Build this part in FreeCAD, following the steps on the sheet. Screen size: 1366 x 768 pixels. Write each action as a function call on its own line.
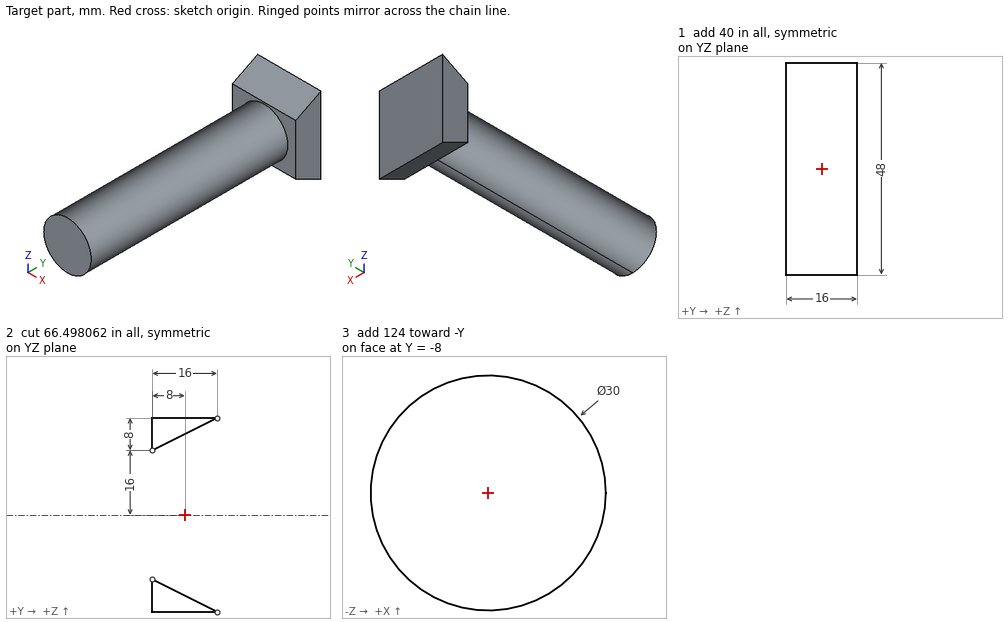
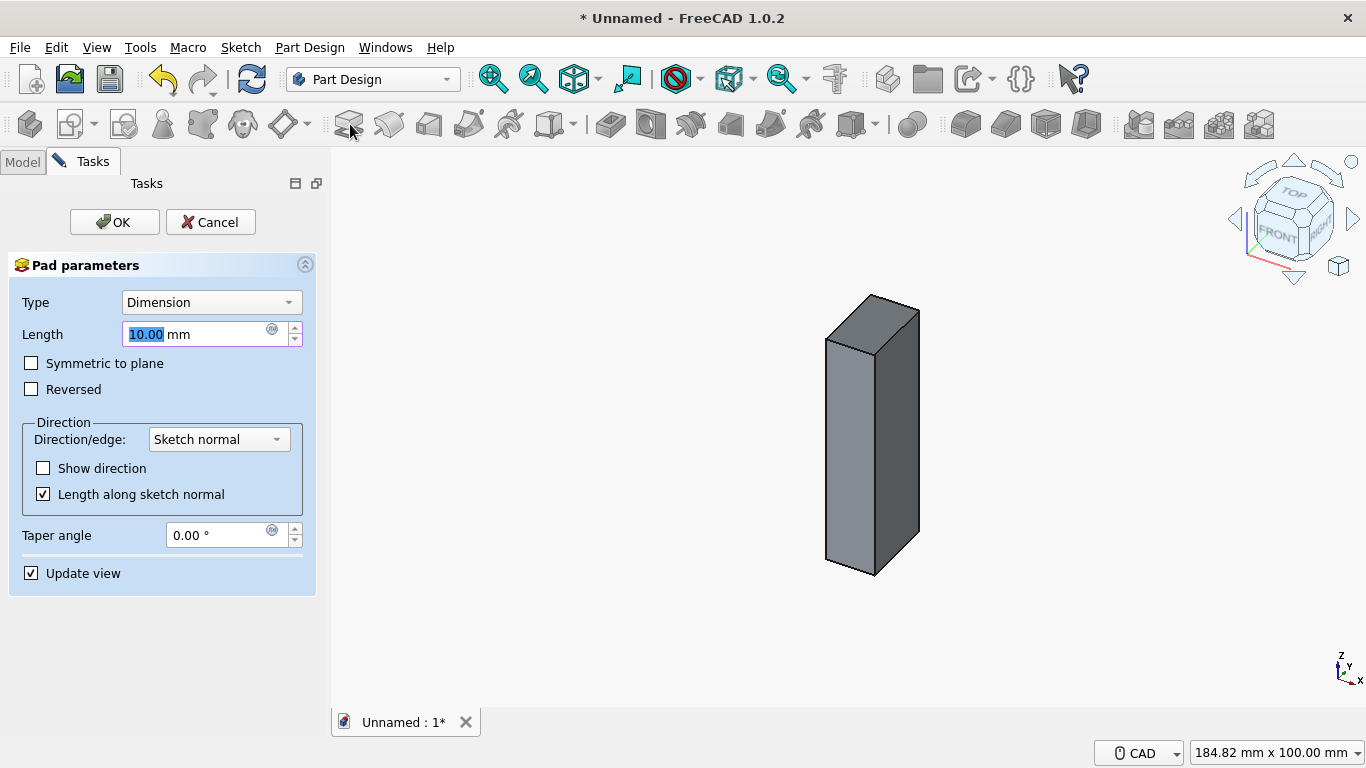
text(40)
key(Tab)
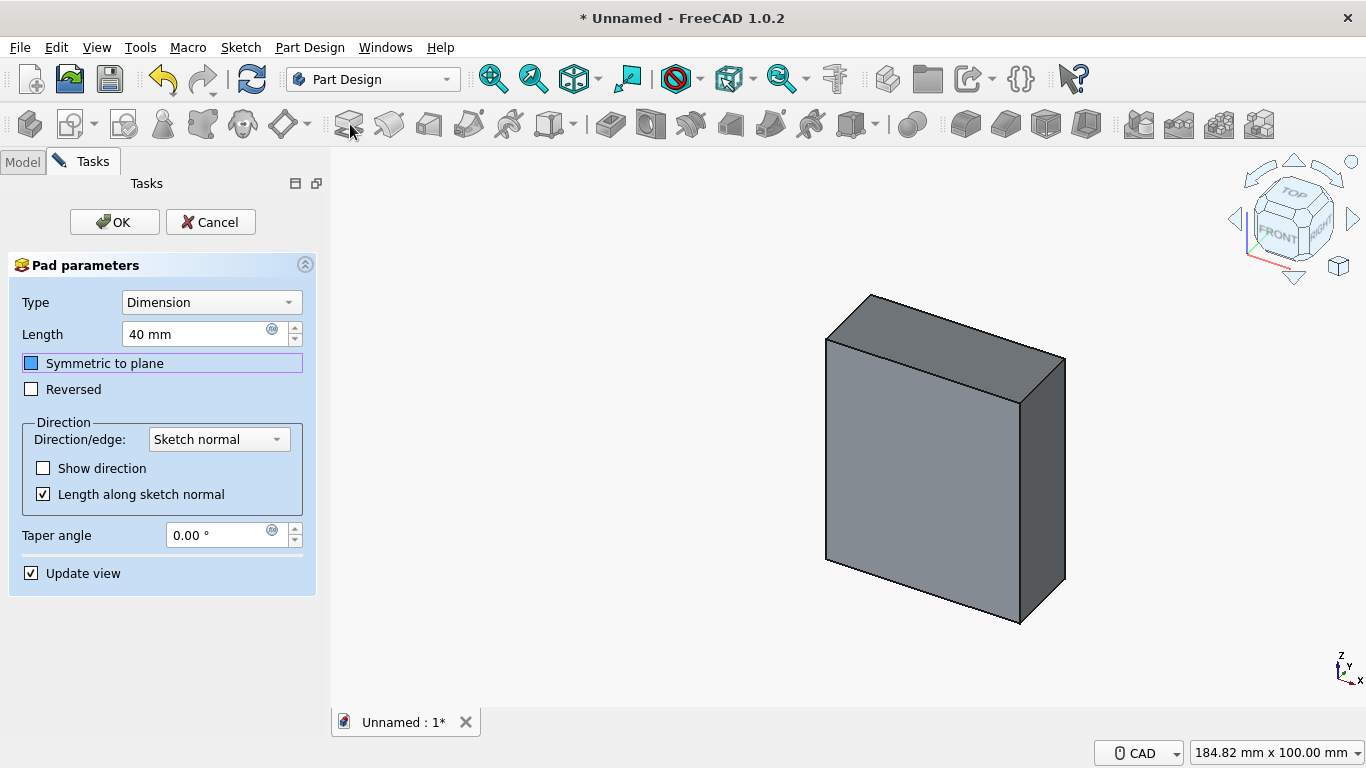
click(30, 363)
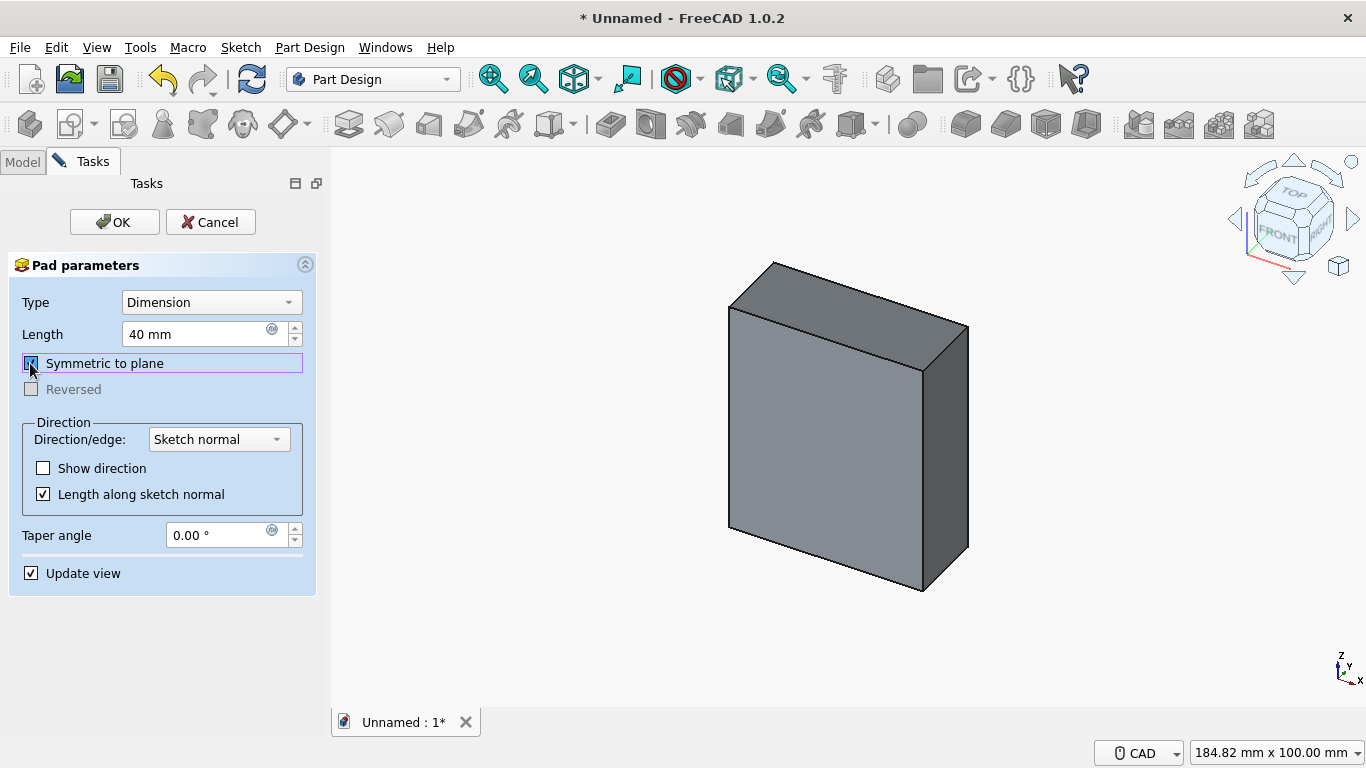
click(115, 222)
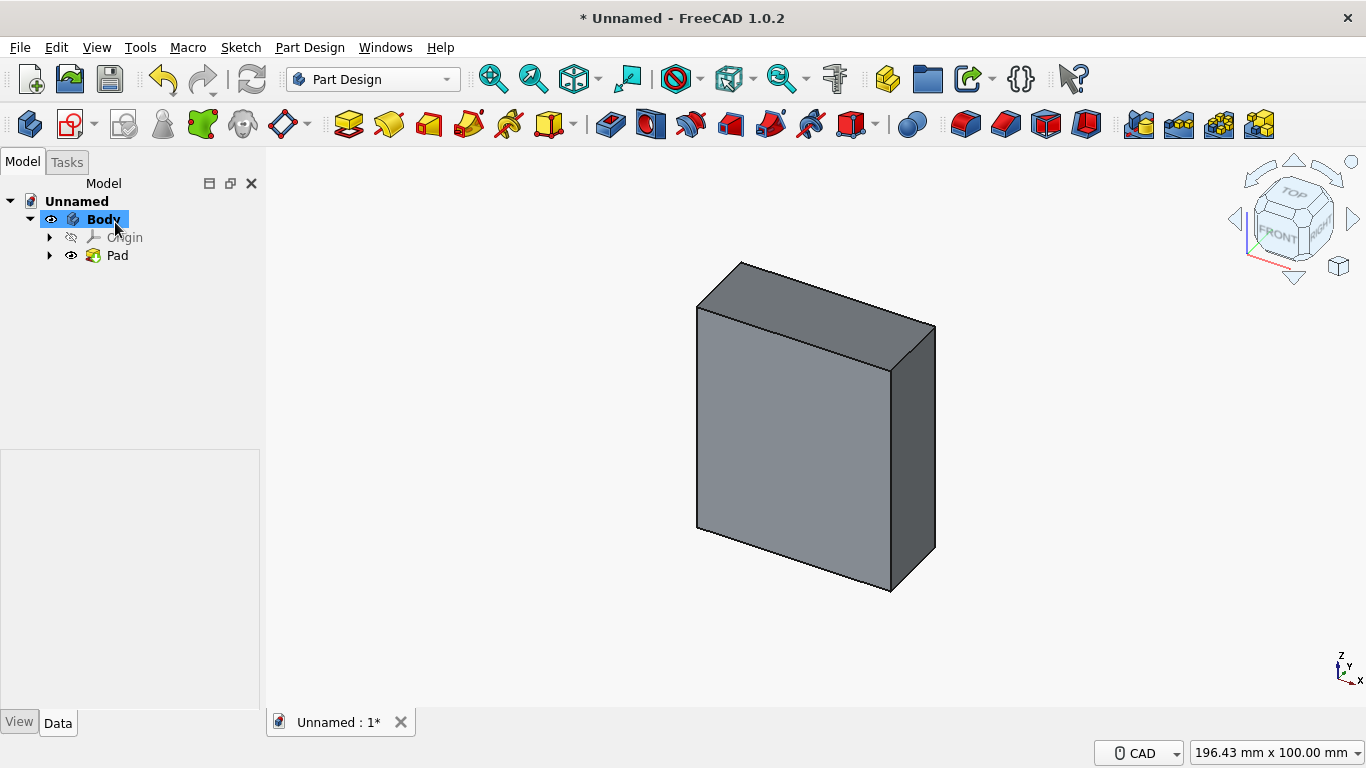
click(70, 124)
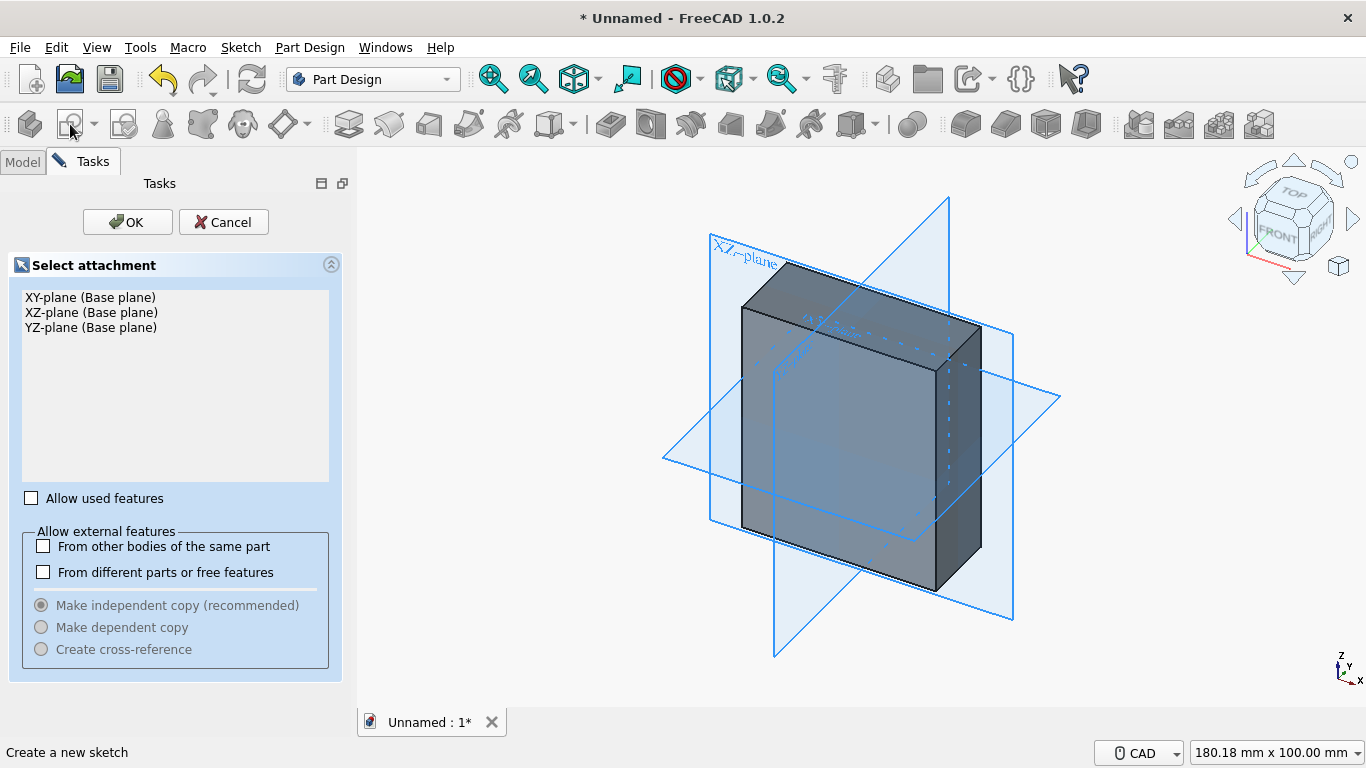
click(82, 328)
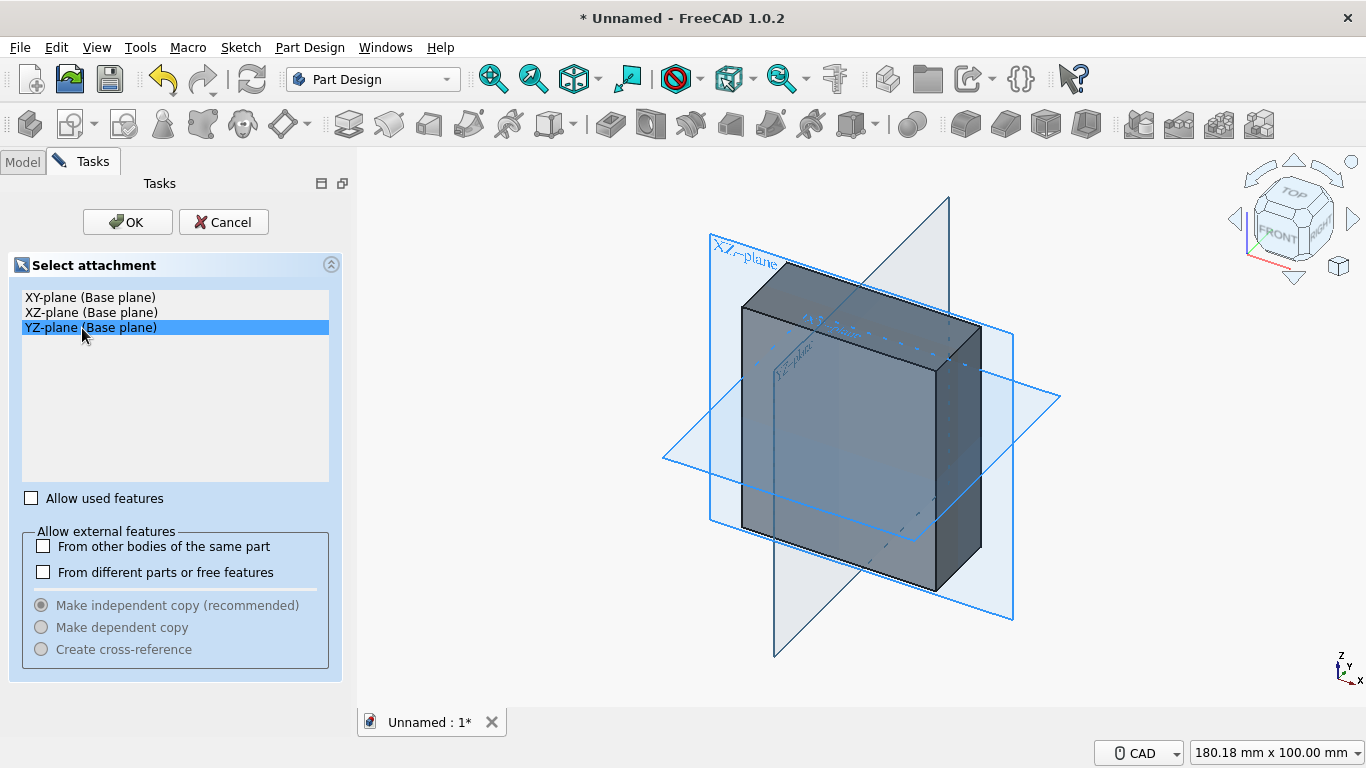
click(128, 222)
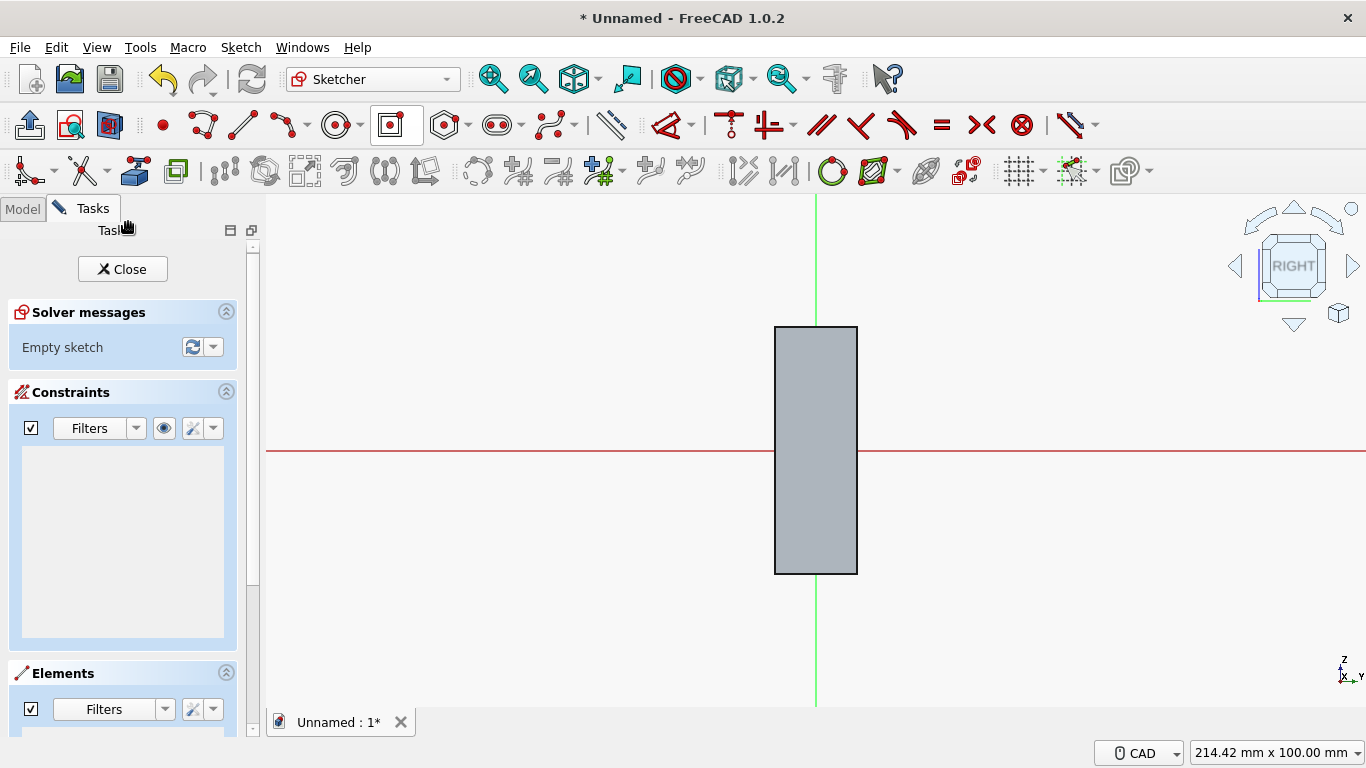
click(110, 126)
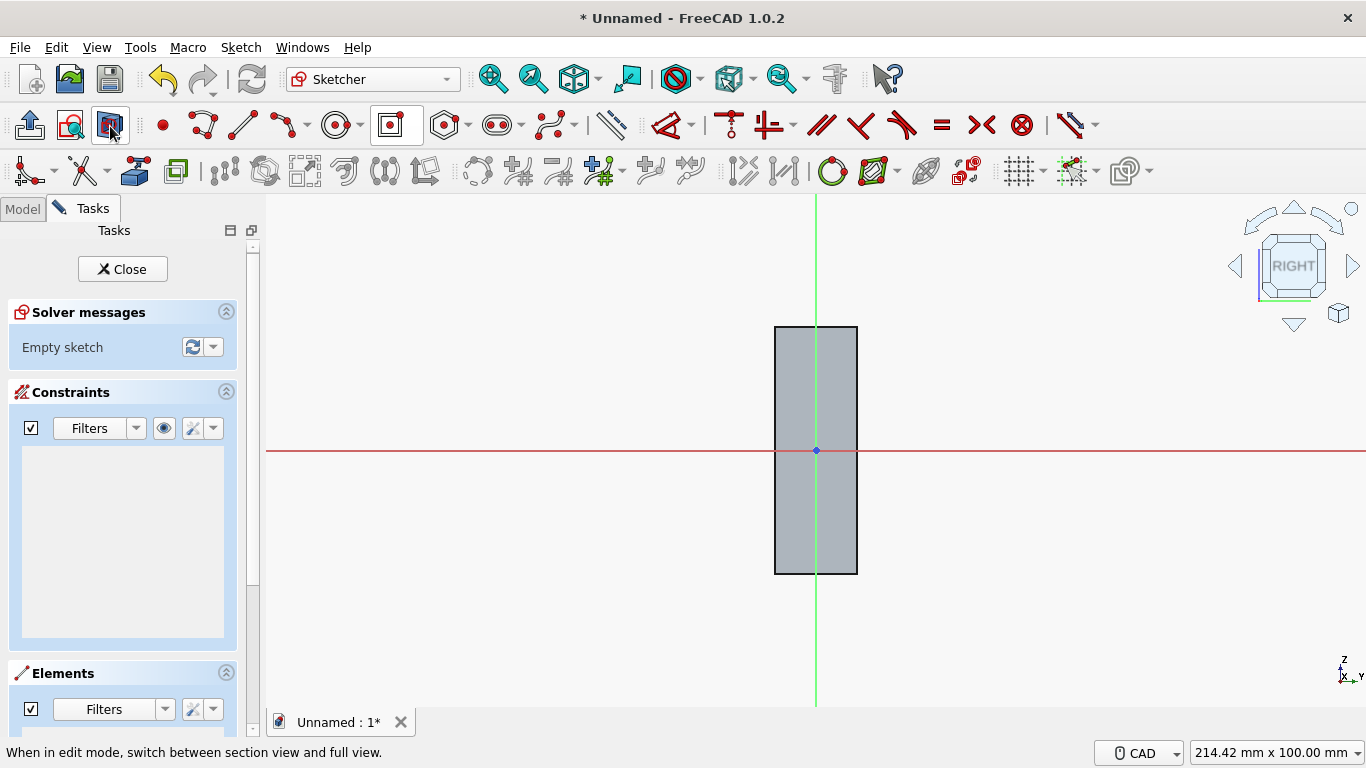
click(204, 126)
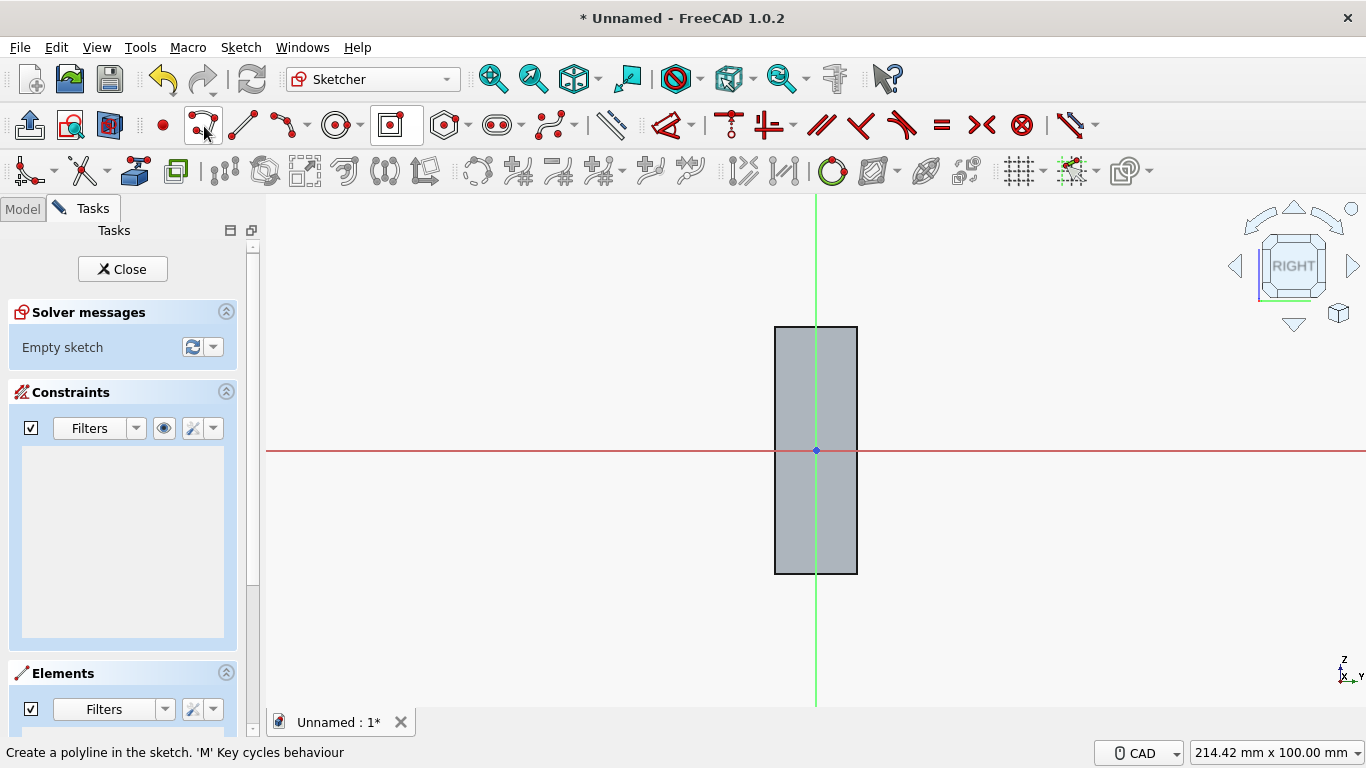
click(775, 368)
click(857, 327)
click(775, 327)
click(775, 369)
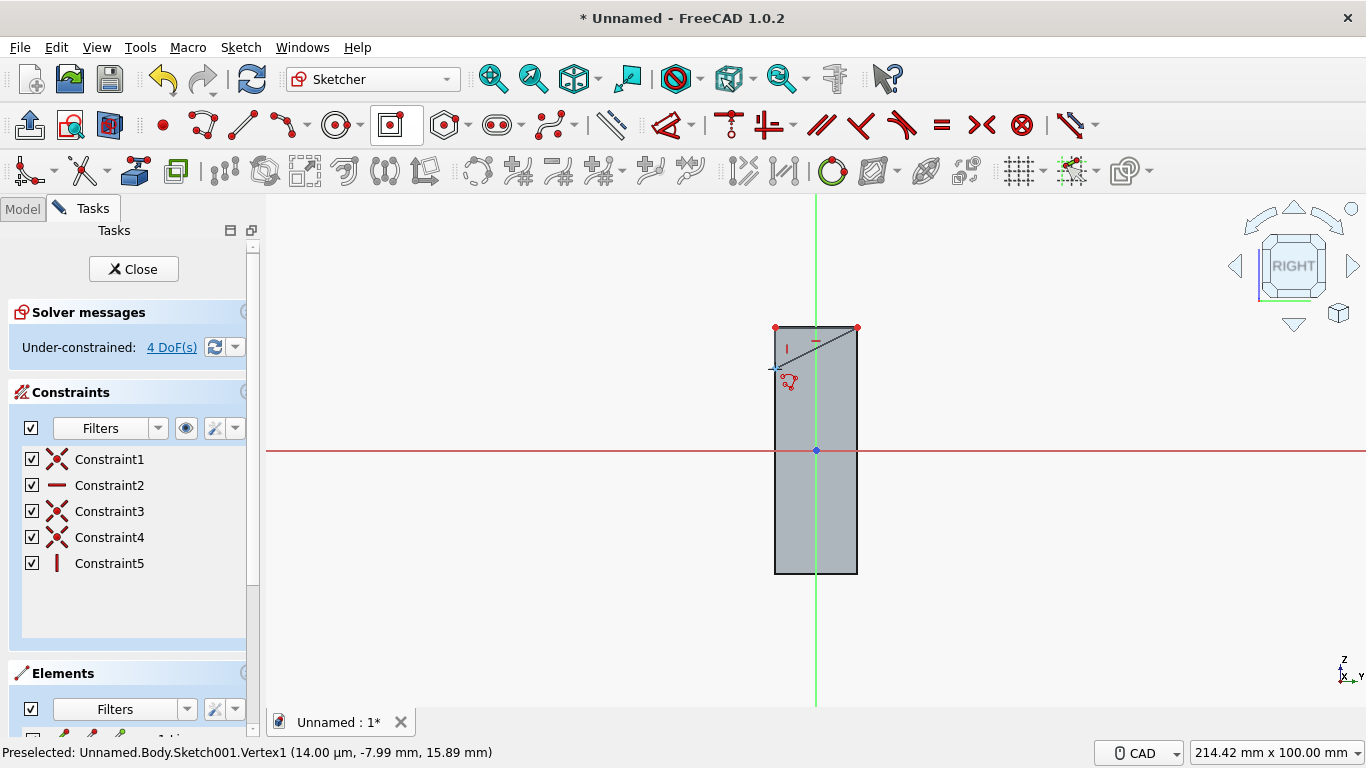
click(775, 533)
click(775, 574)
click(857, 574)
click(775, 534)
key(Escape)
key(Escape)